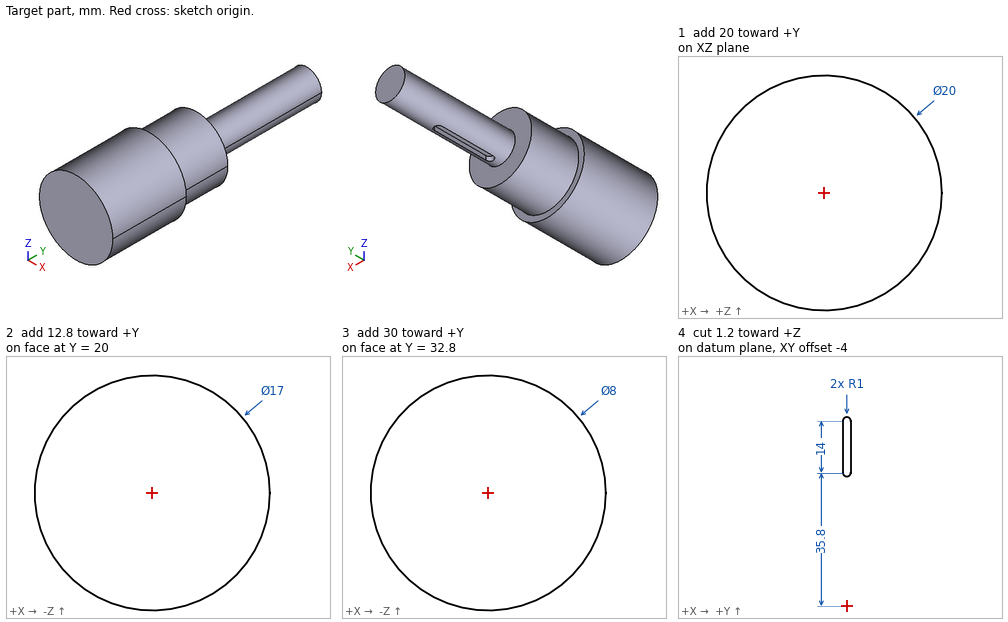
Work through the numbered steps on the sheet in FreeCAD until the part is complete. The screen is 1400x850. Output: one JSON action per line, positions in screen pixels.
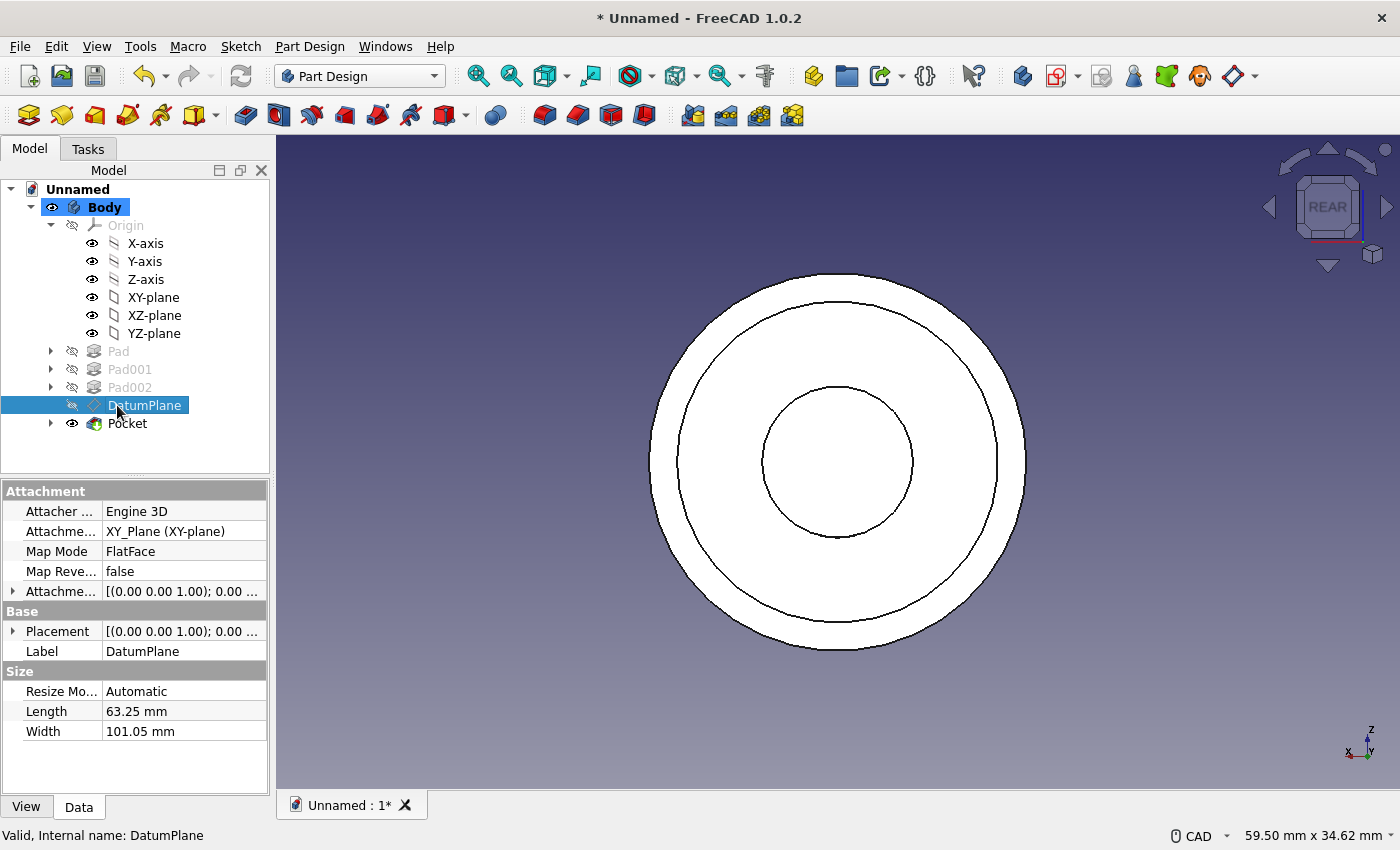
{"action": "key", "text": "0"}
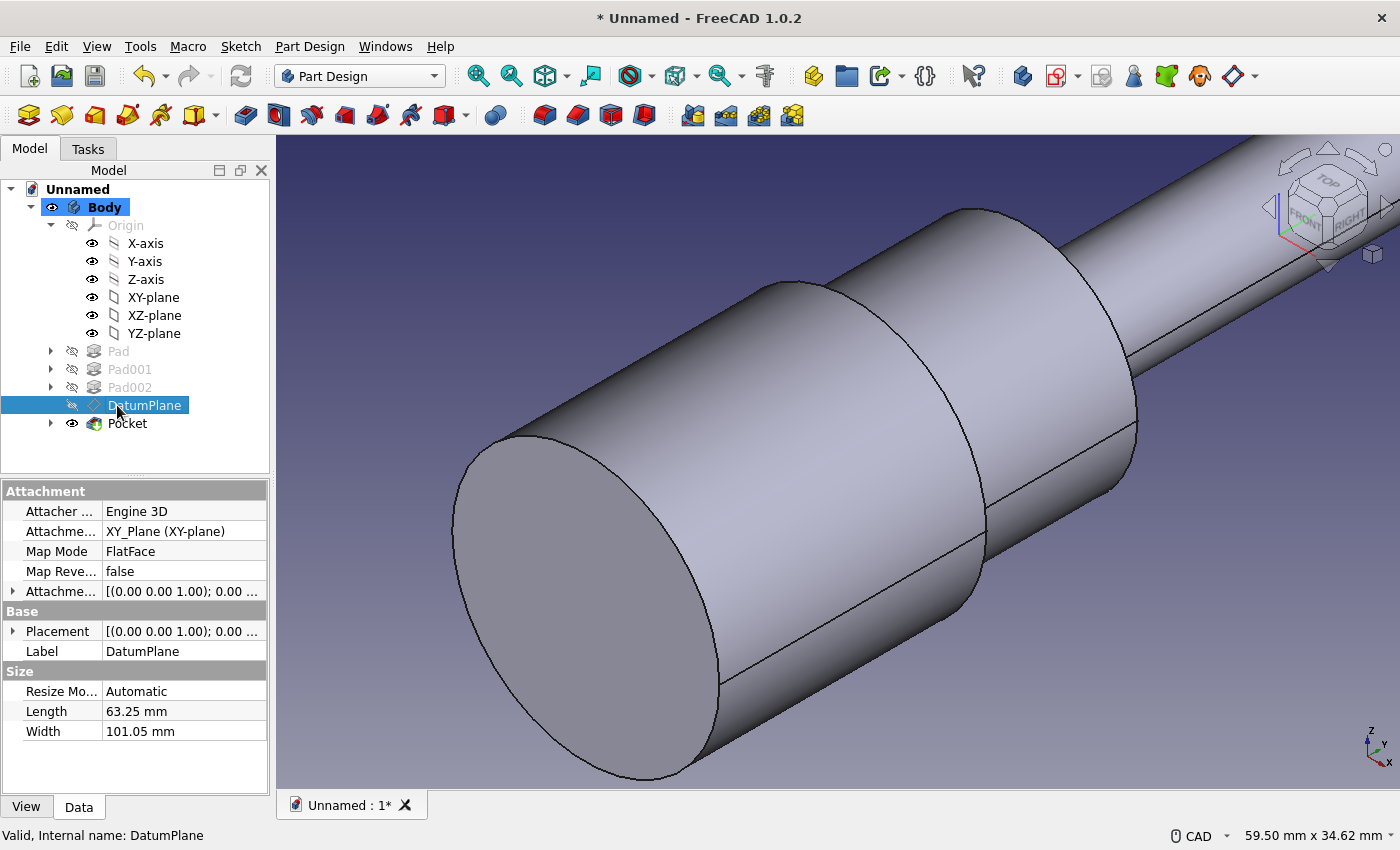
{"action": "left_click", "coordinate": [479, 76]}